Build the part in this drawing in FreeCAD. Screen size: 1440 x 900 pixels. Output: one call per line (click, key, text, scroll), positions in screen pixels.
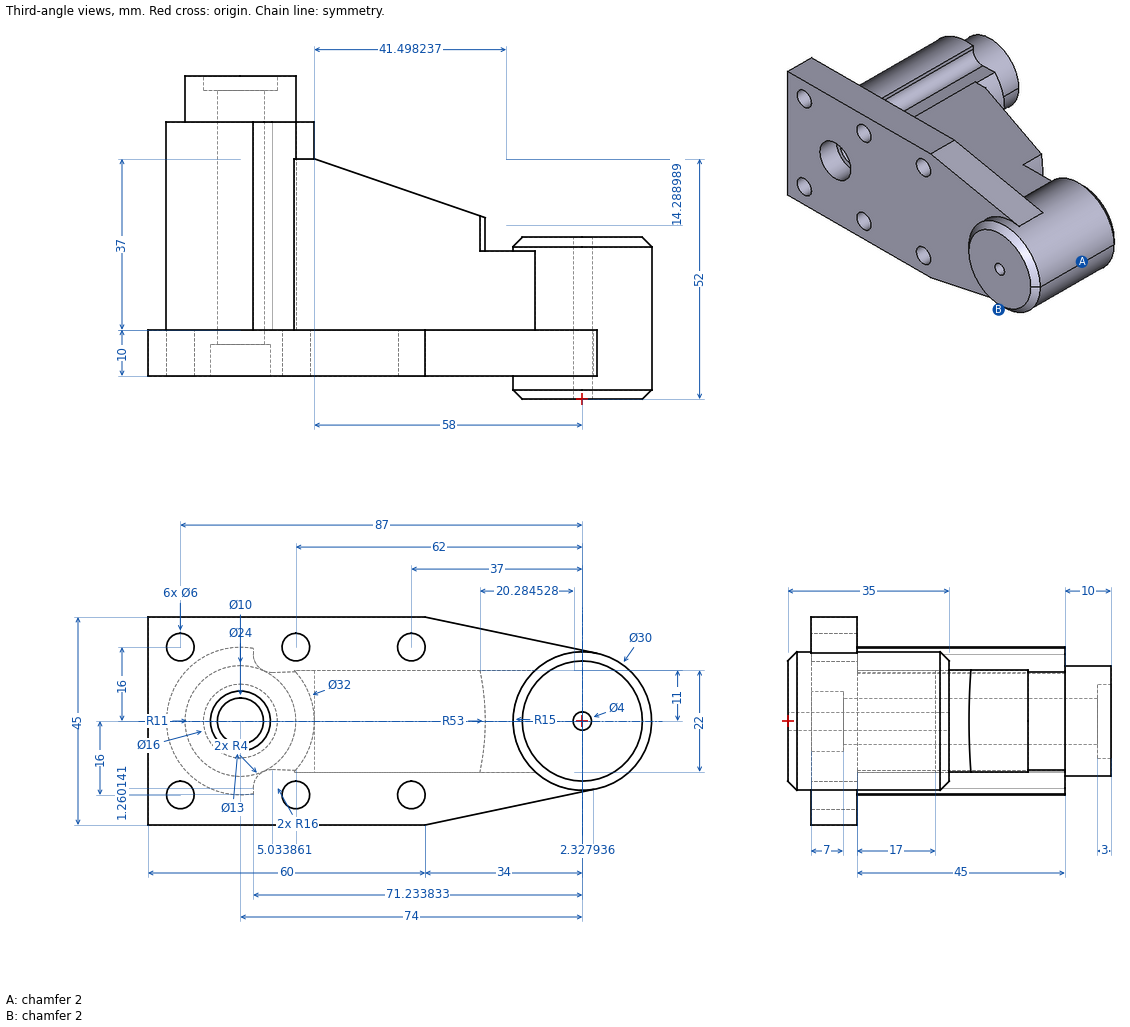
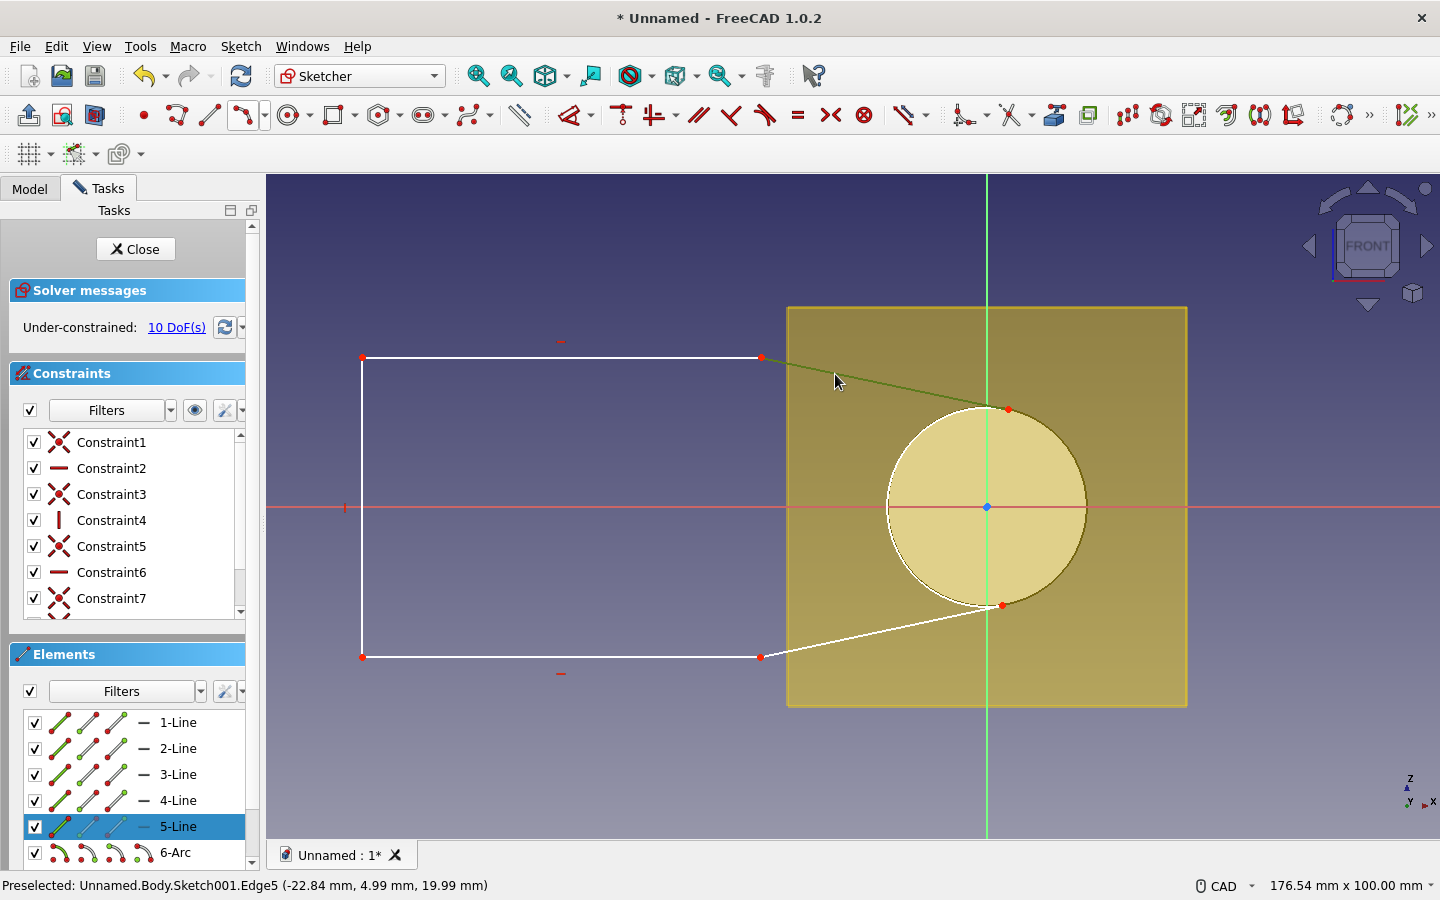
click(913, 441)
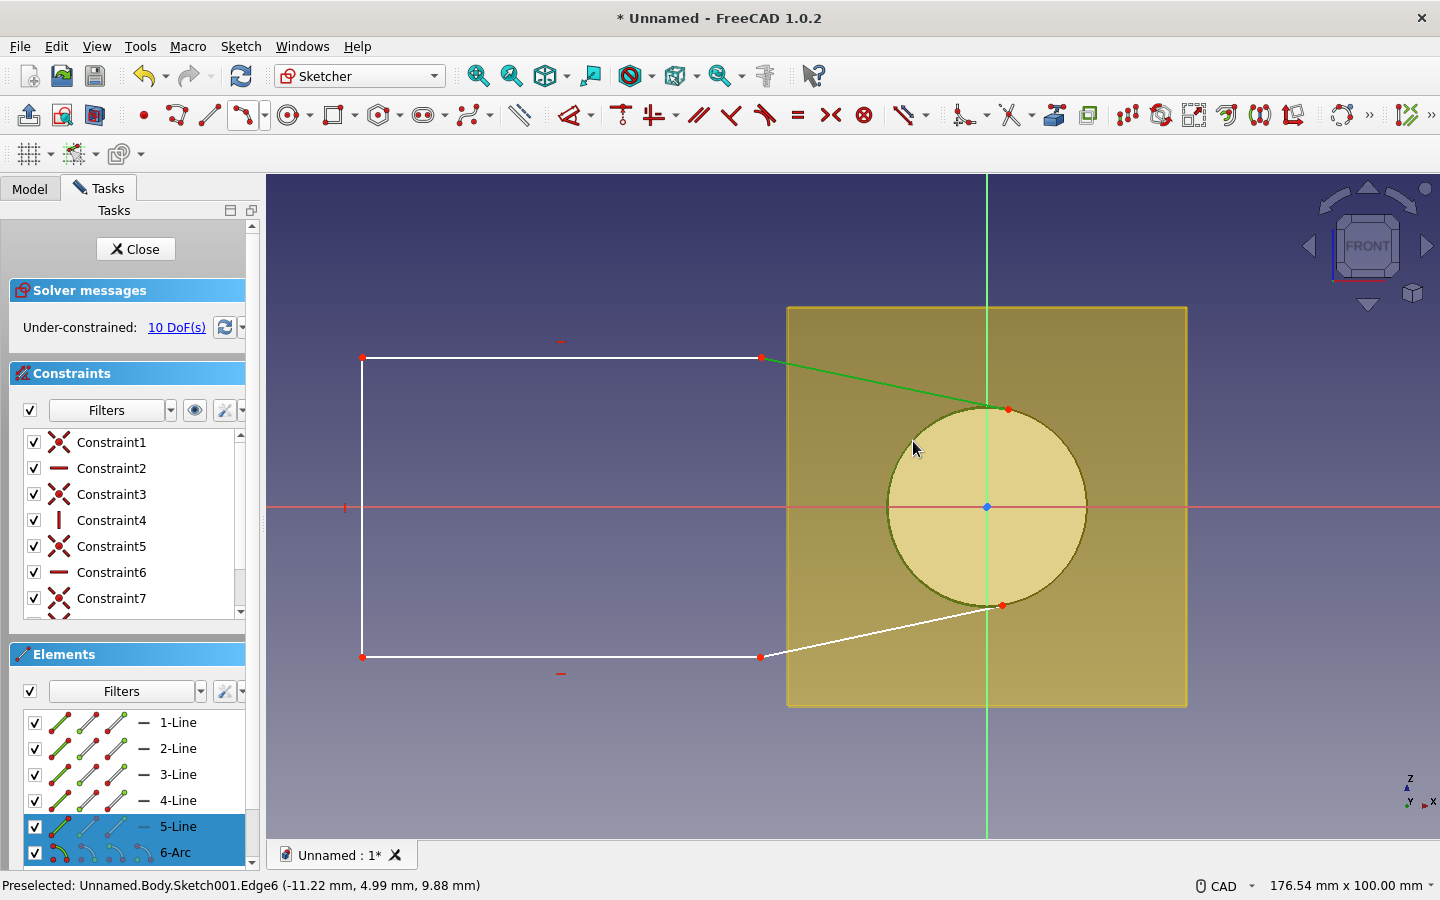
click(765, 116)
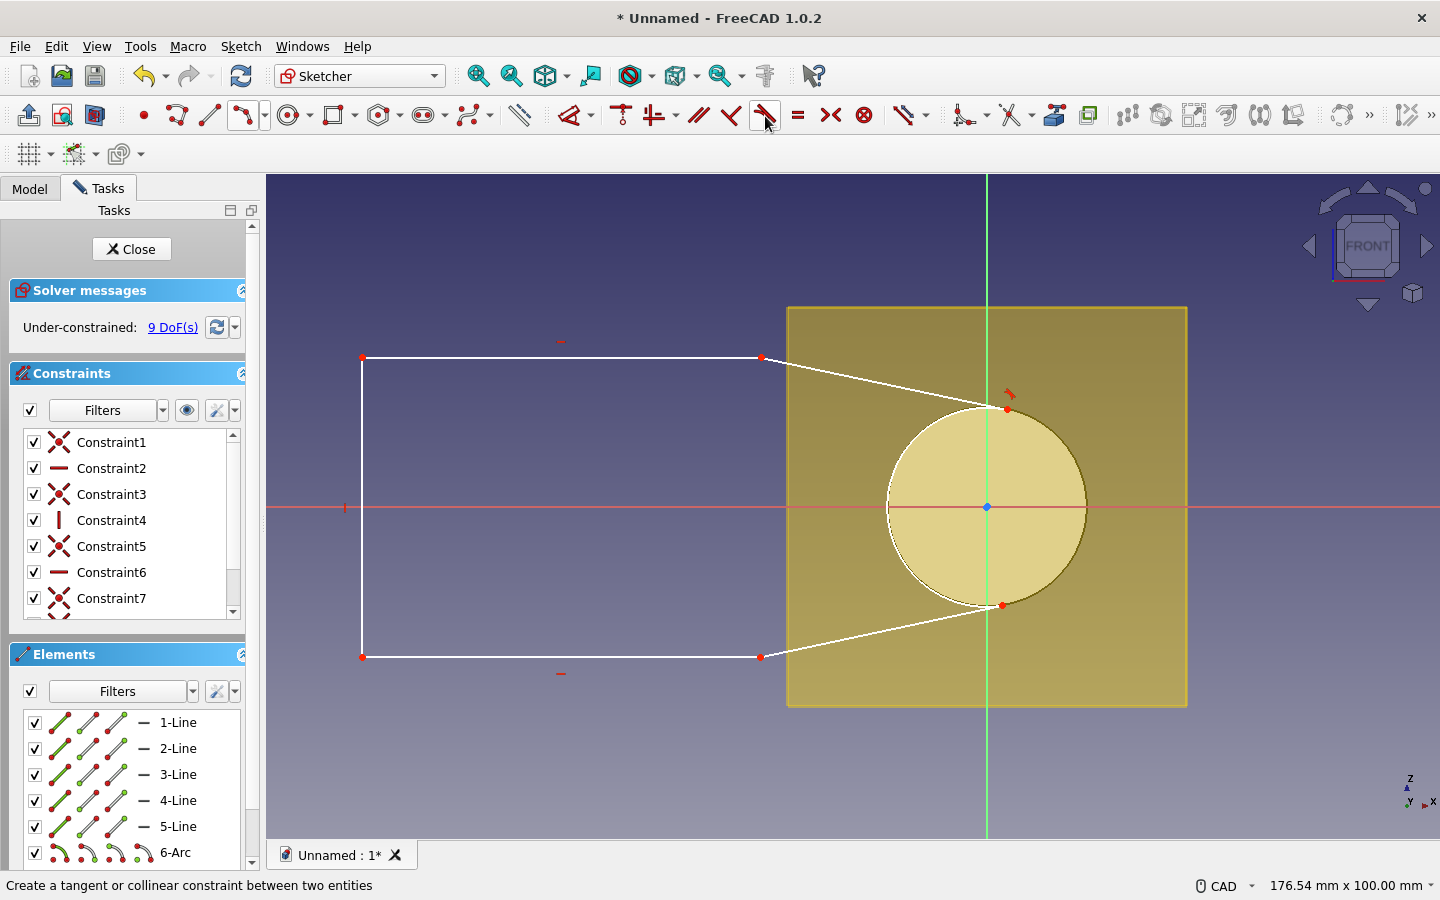
drag(977, 497, 997, 517)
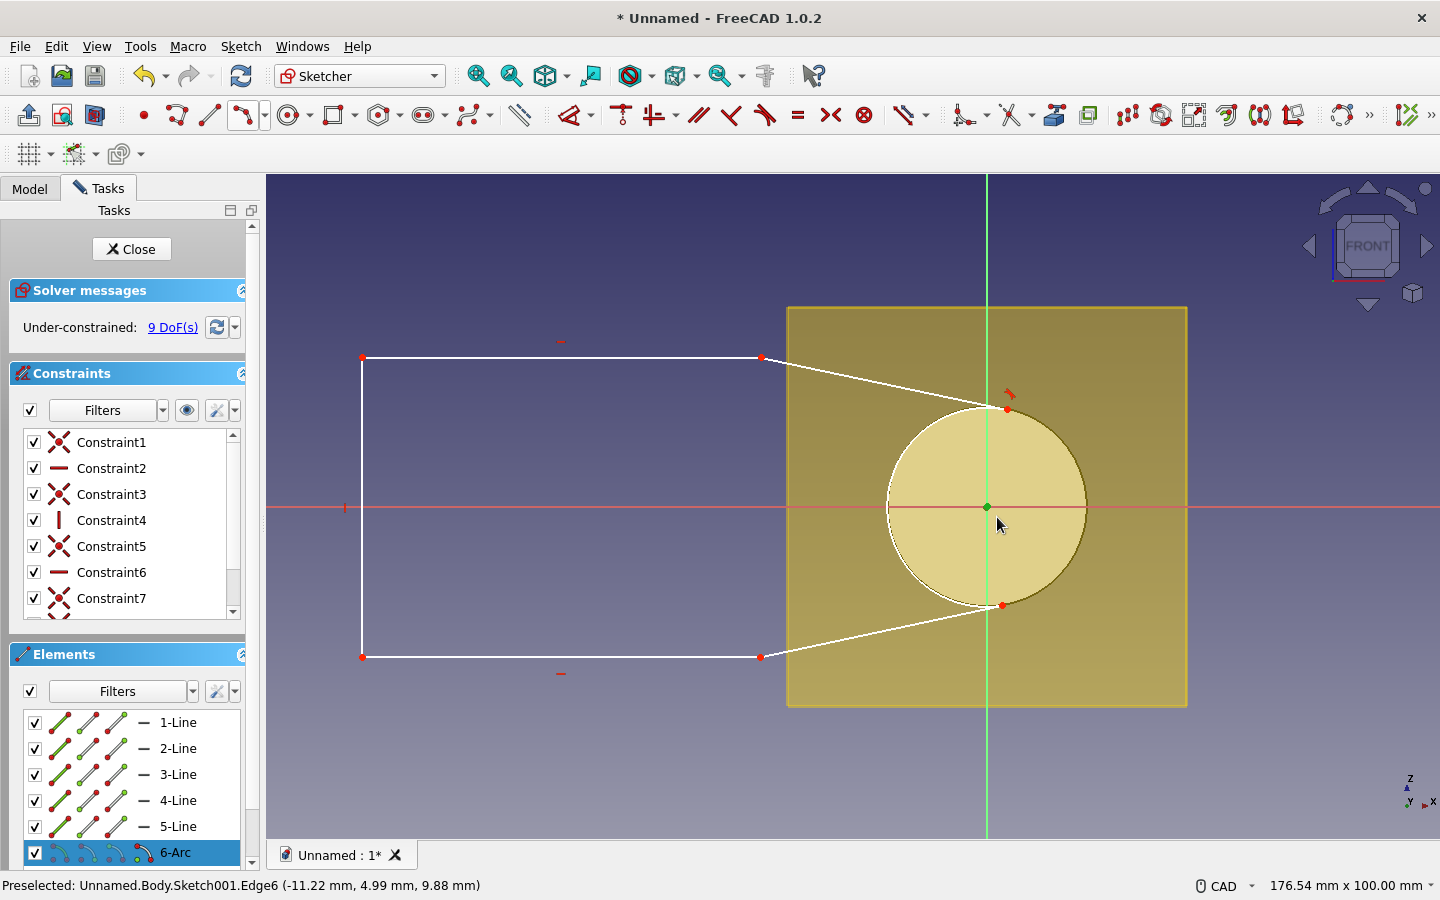
click(621, 116)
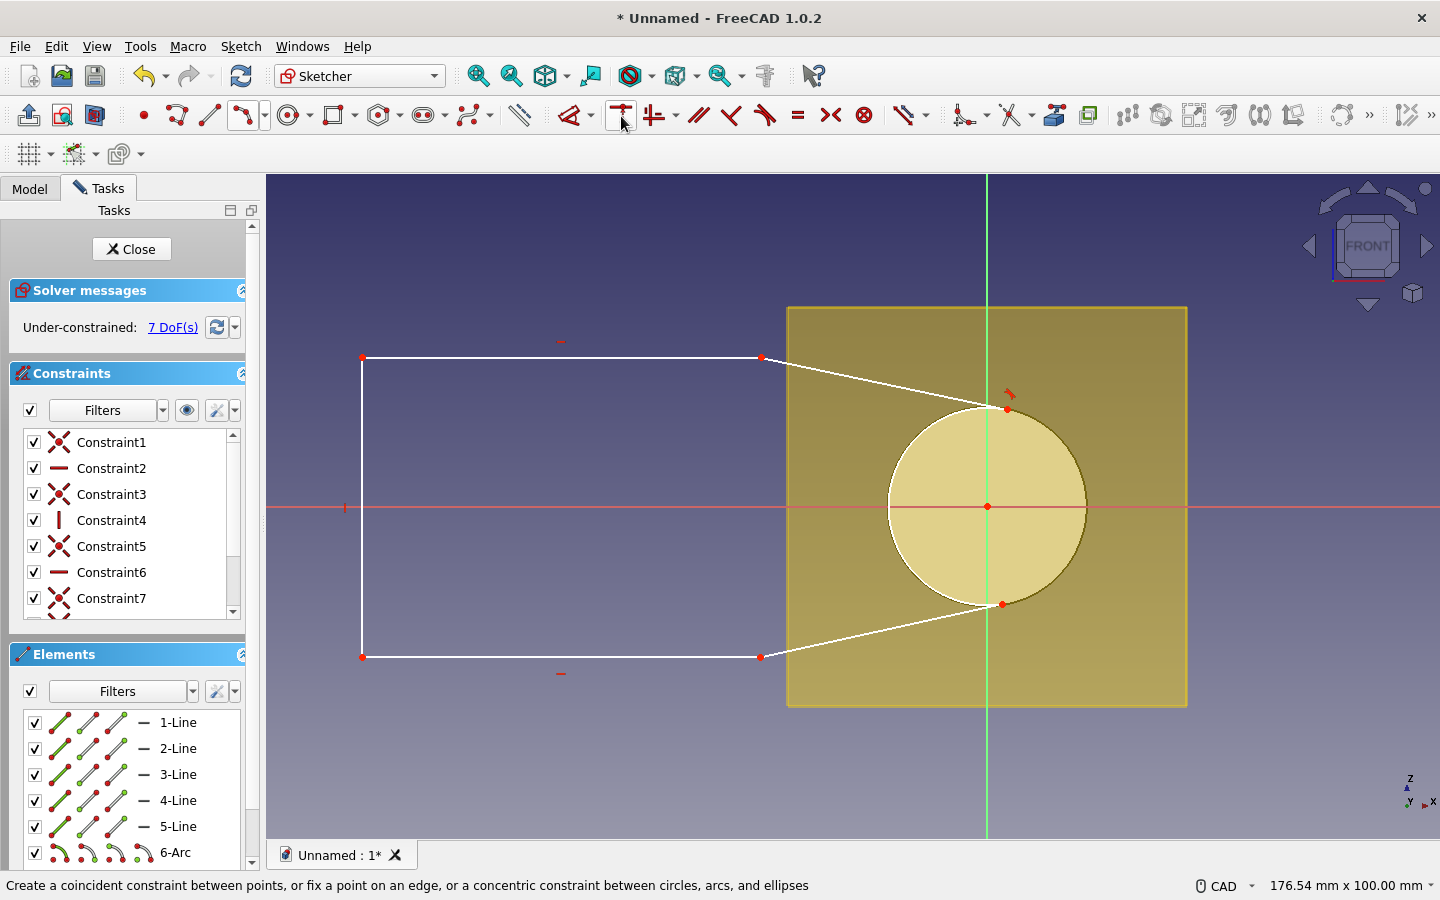
click(761, 657)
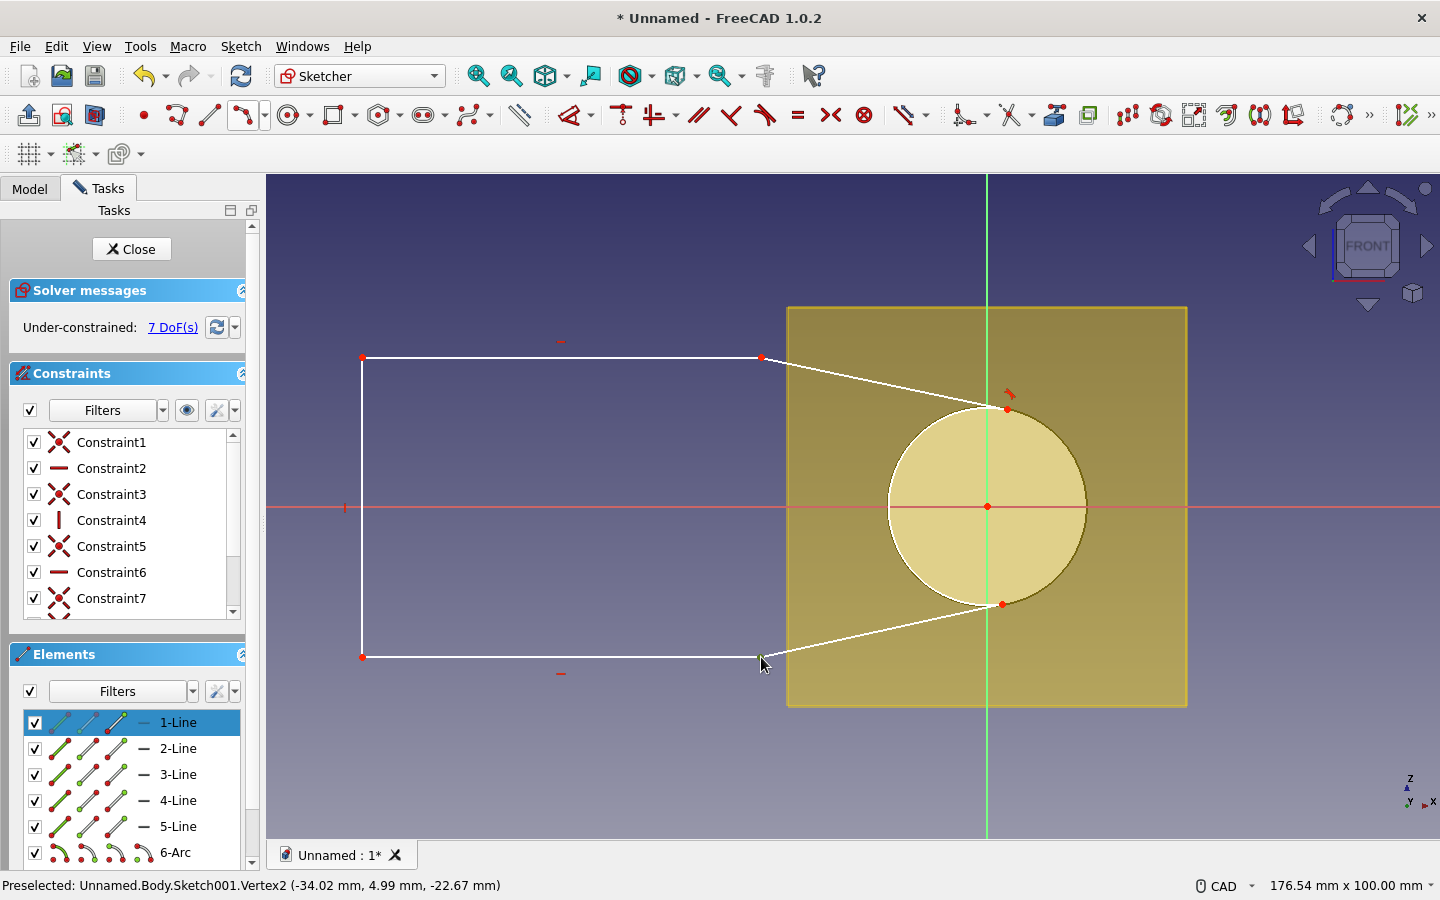
click(761, 358)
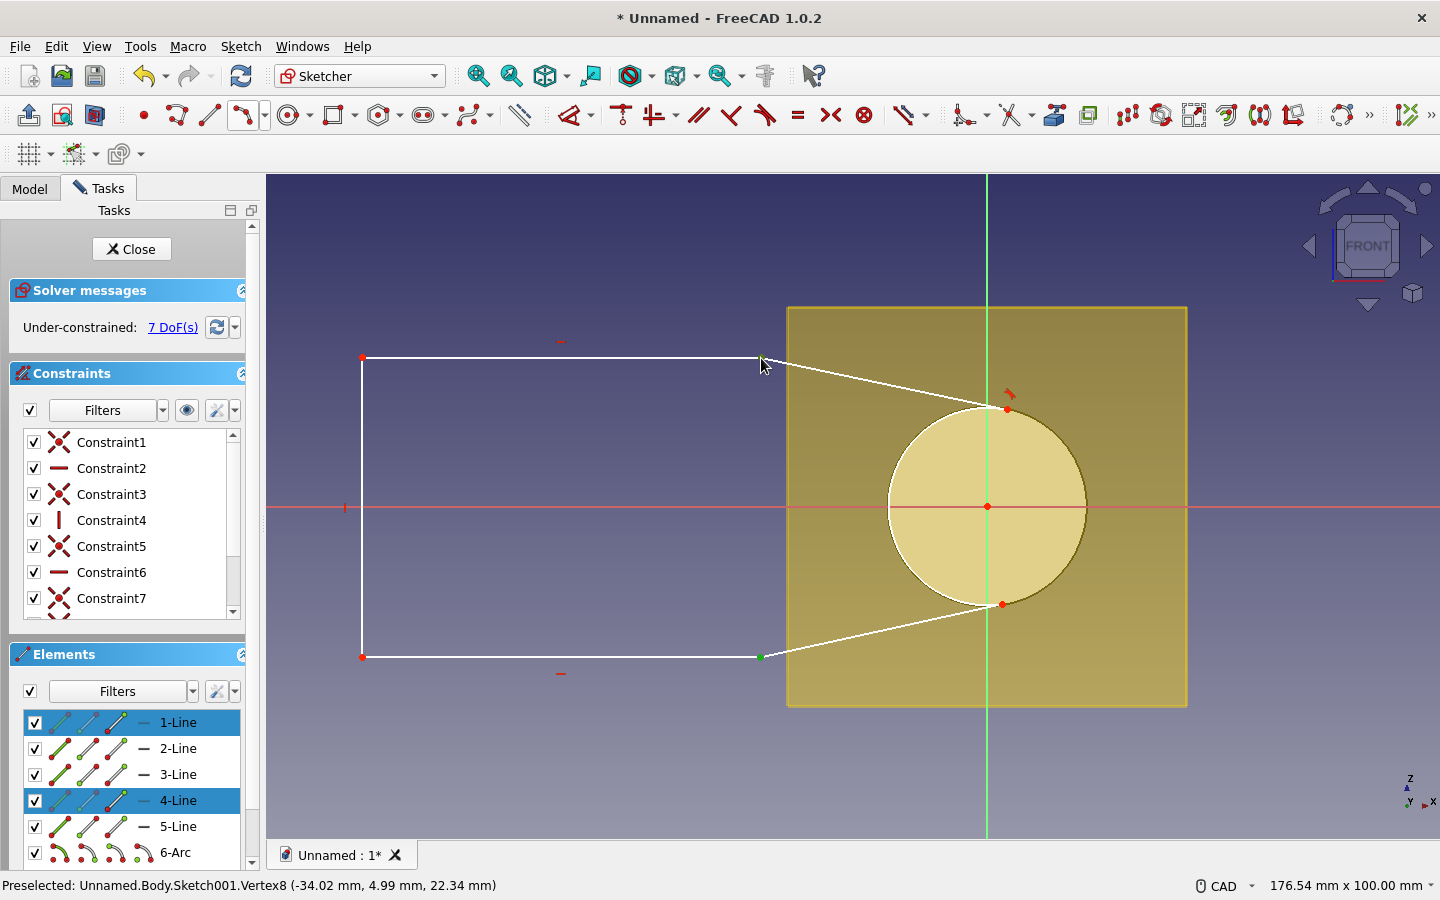
click(434, 507)